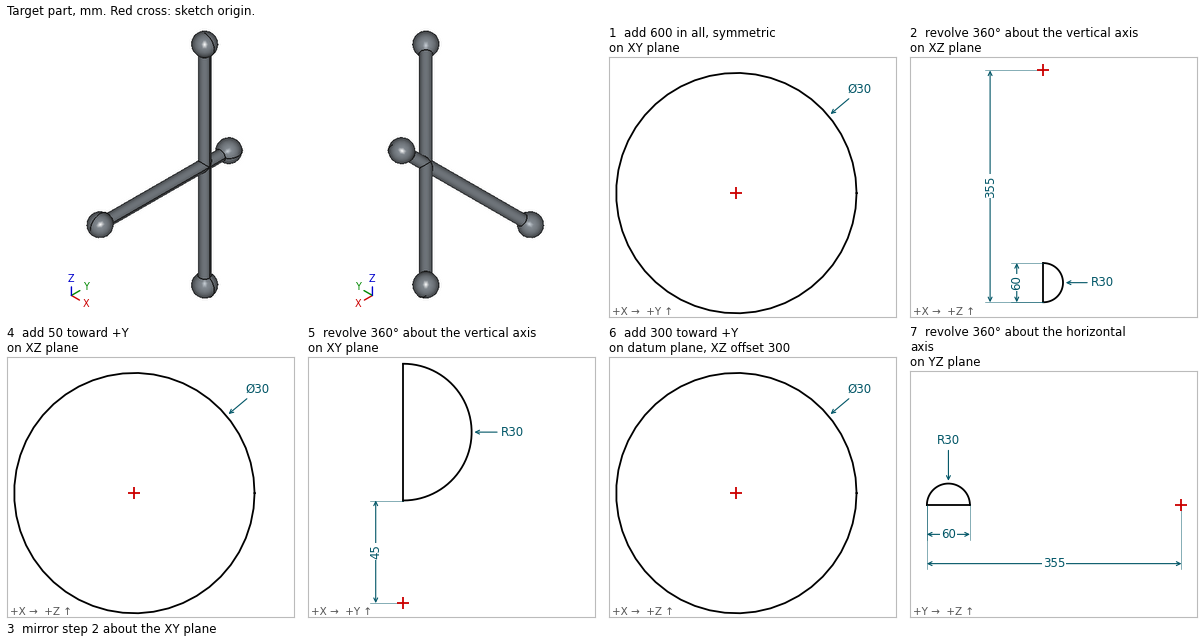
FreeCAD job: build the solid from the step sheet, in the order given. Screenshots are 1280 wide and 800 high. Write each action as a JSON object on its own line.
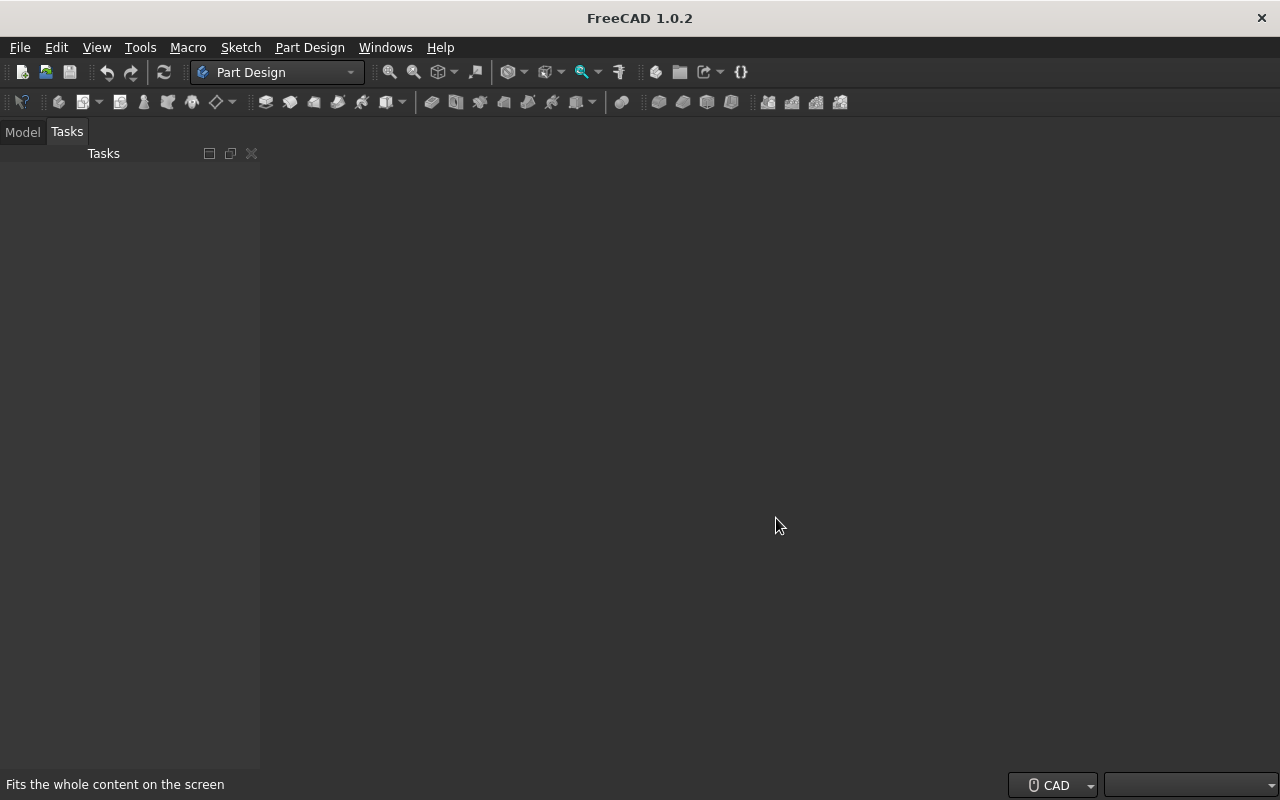
{"action": "key", "text": "ctrl+n"}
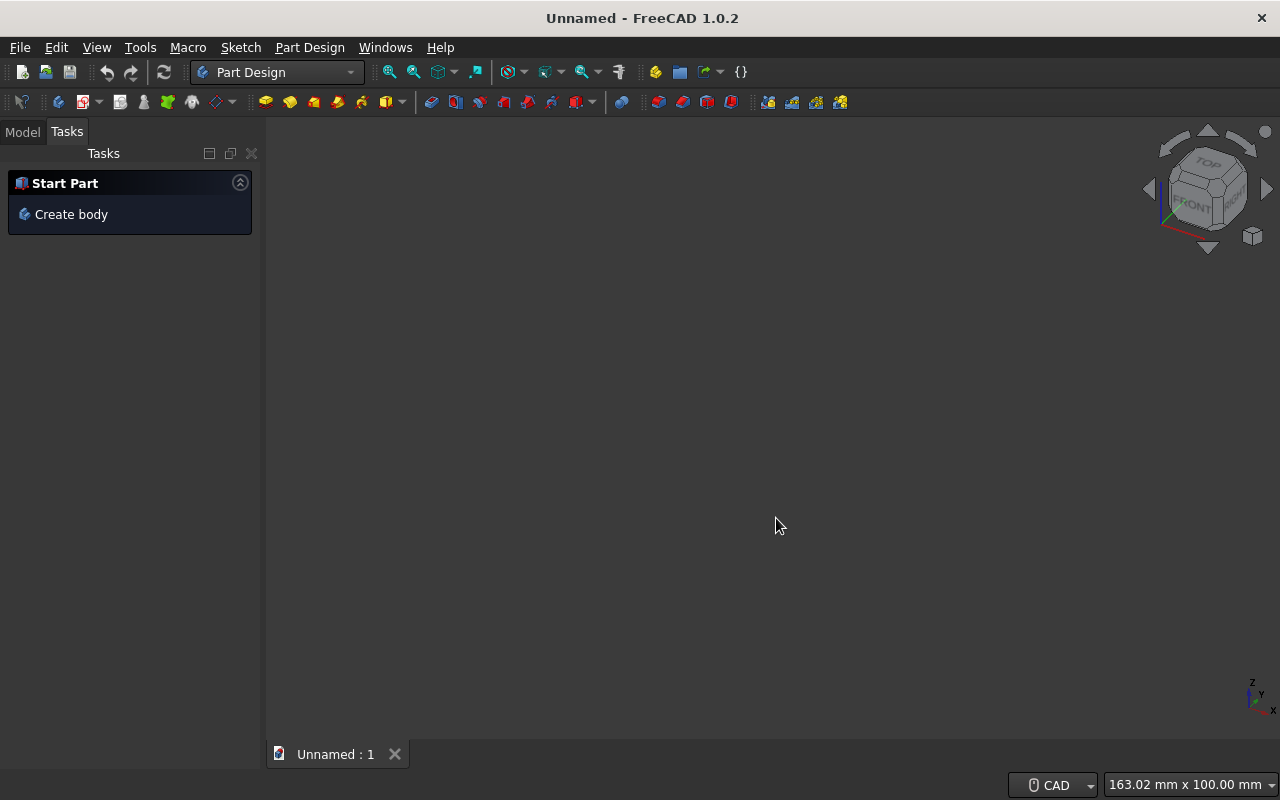
{"action": "left_click", "coordinate": [84, 102]}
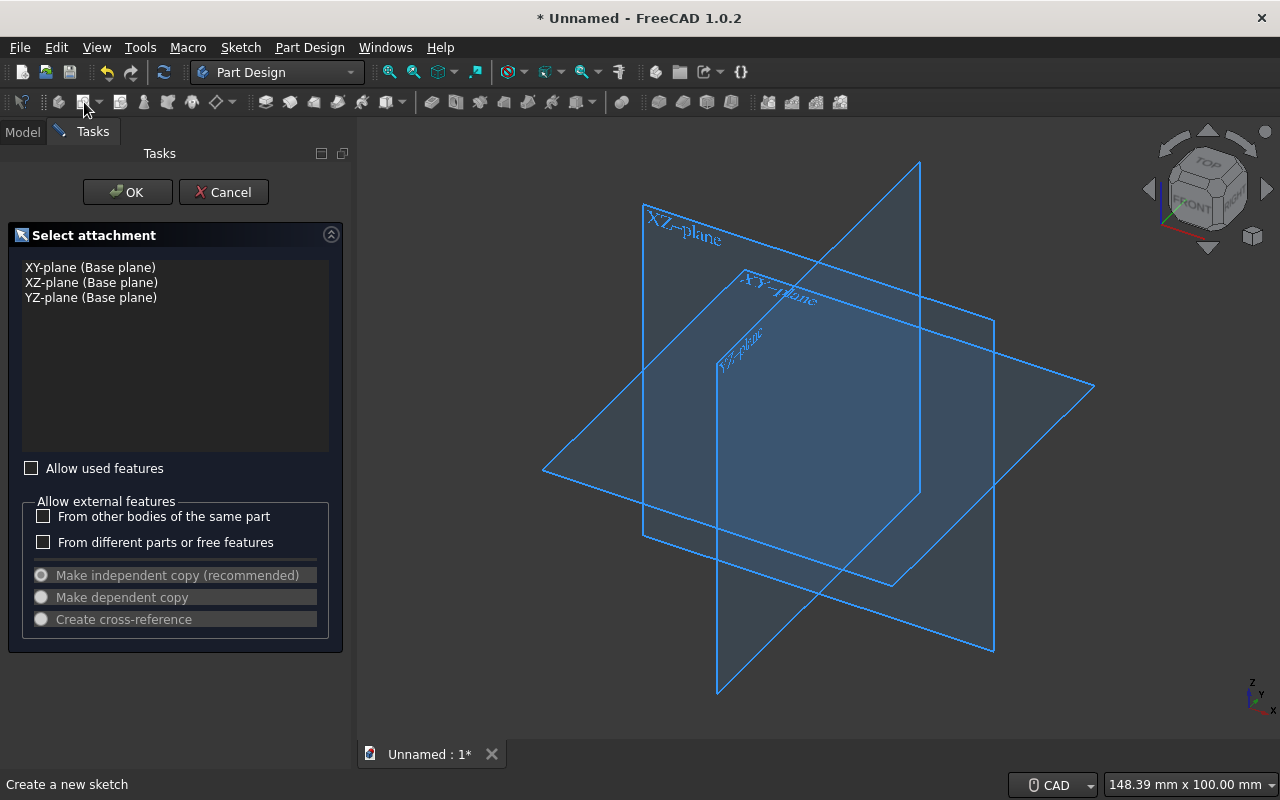
{"action": "left_click", "coordinate": [82, 268]}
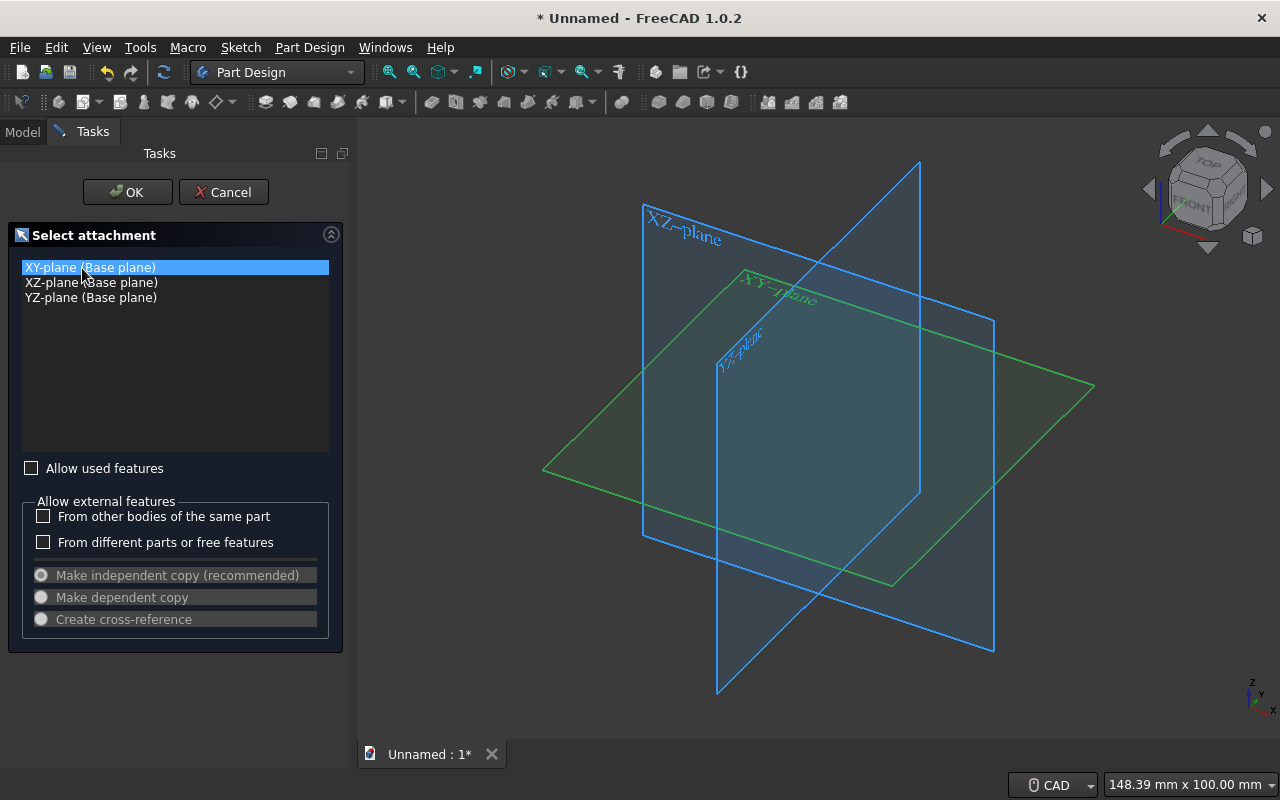
{"action": "left_click", "coordinate": [128, 192]}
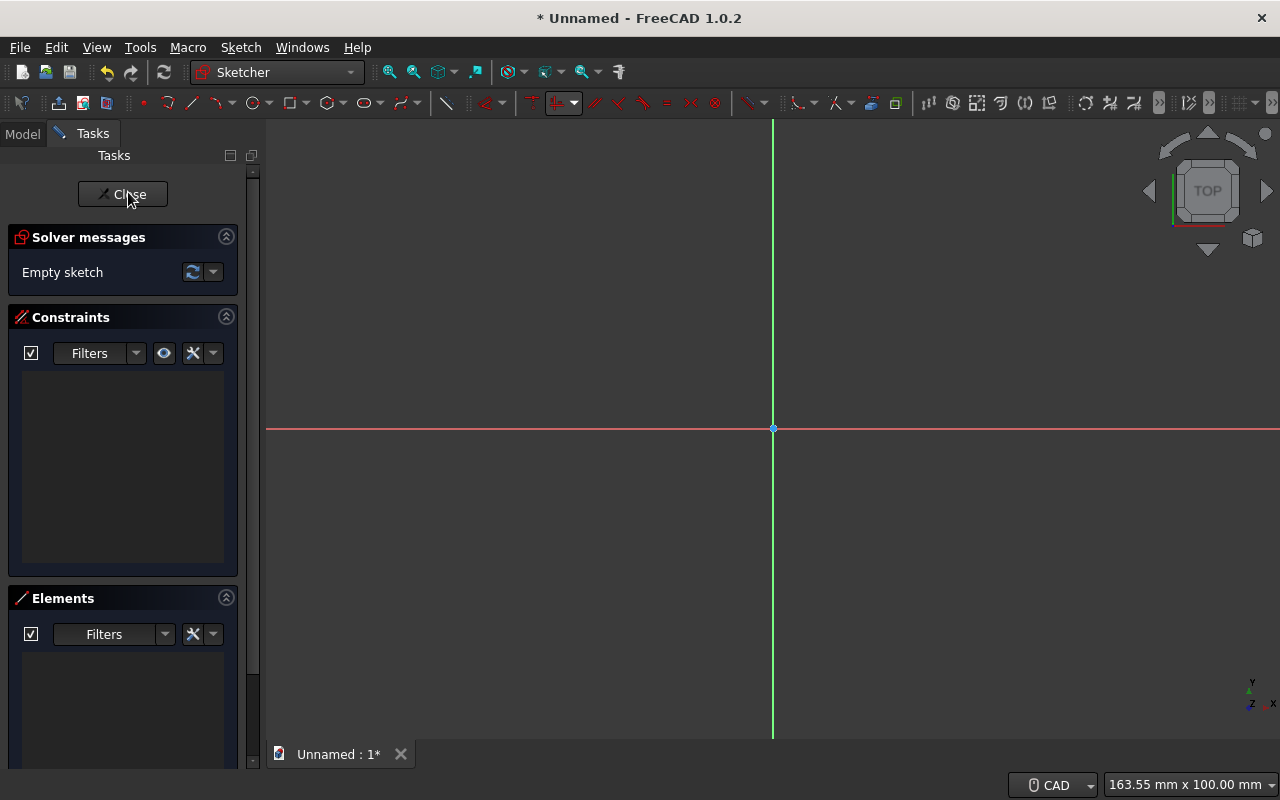
{"action": "scroll", "coordinate": [829, 429], "scroll_direction": "up", "scroll_amount": 4}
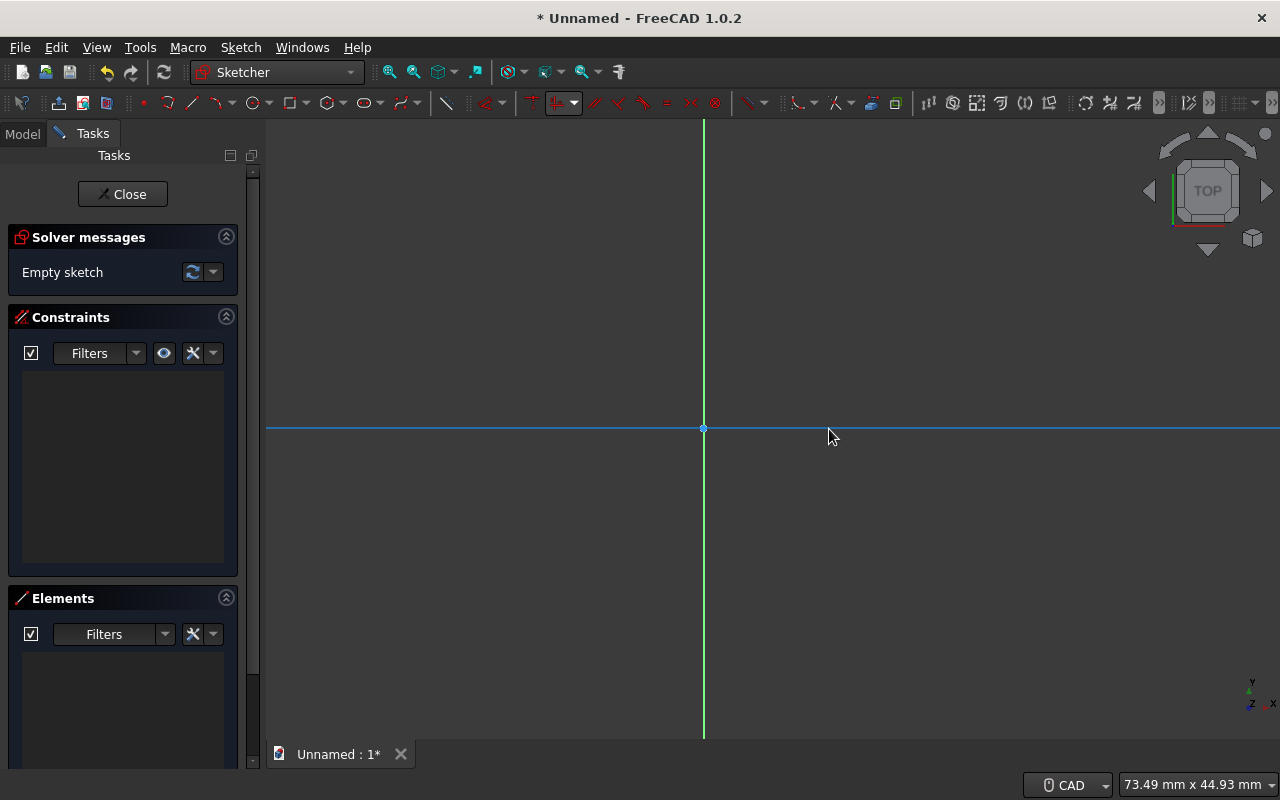
{"action": "left_click", "coordinate": [254, 104]}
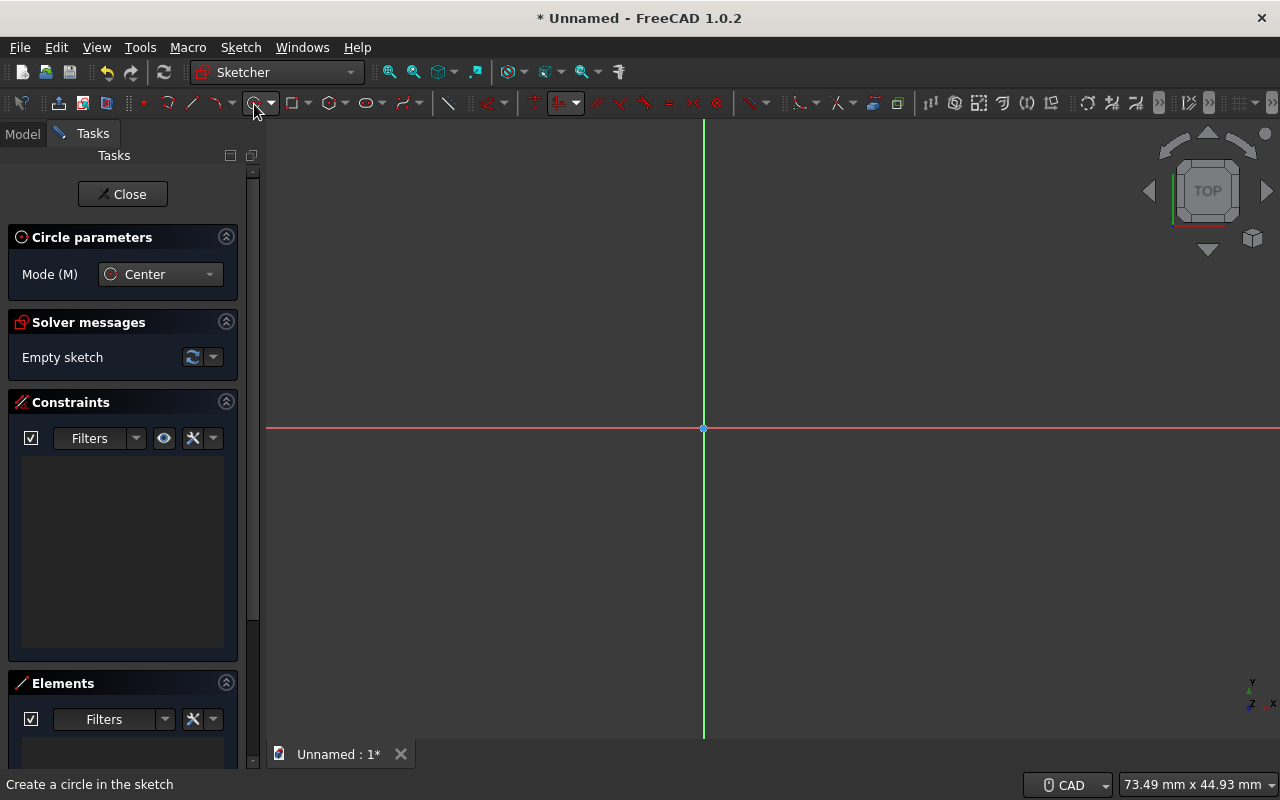
{"action": "left_click", "coordinate": [704, 428]}
{"action": "left_click", "coordinate": [850, 282]}
{"action": "key", "text": "Escape"}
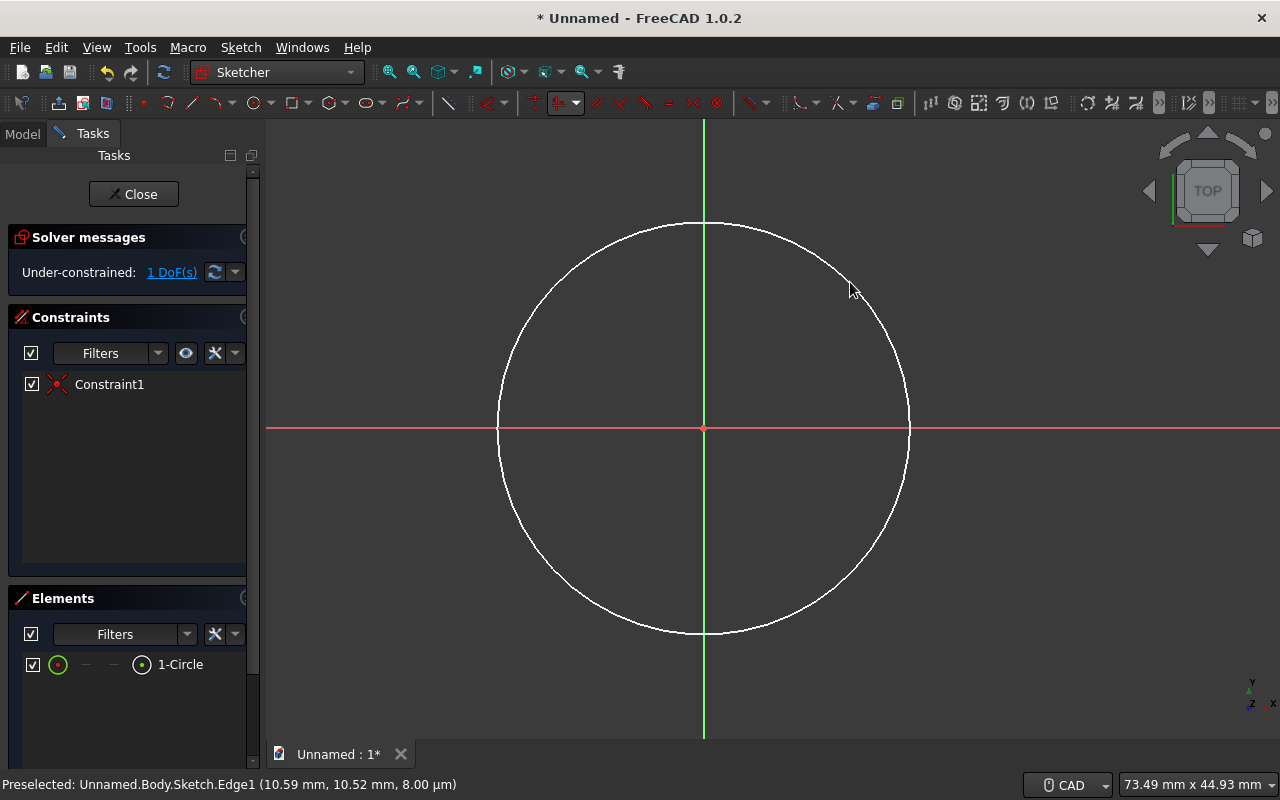
{"action": "left_click", "coordinate": [849, 282]}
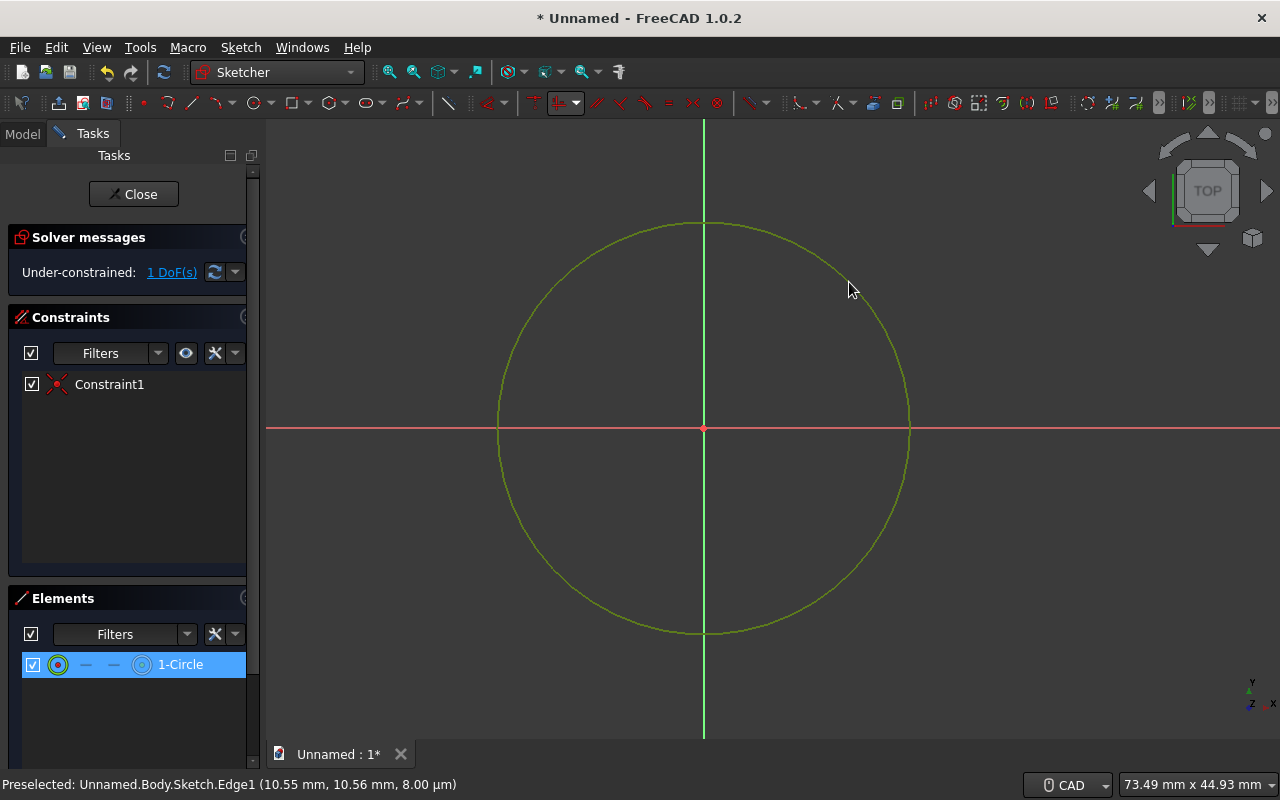
{"action": "key", "text": "k o"}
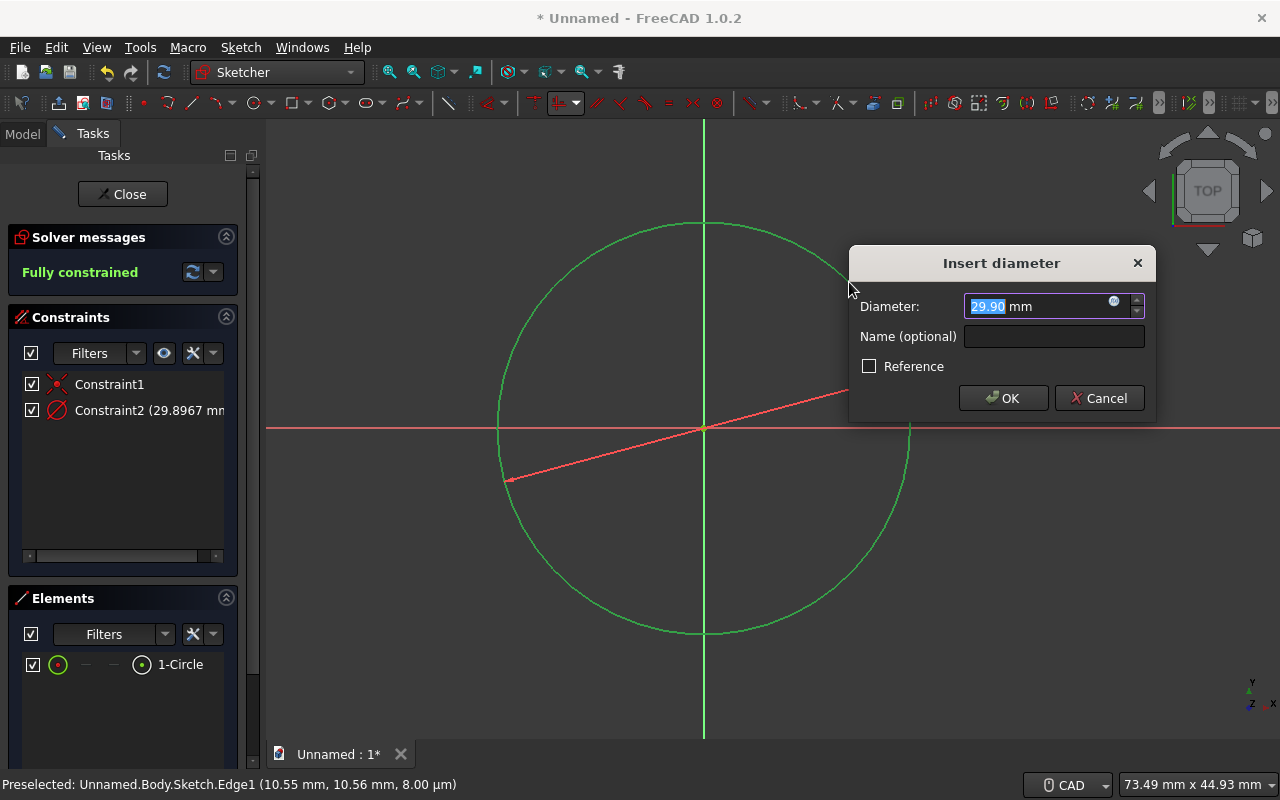
{"action": "type", "text": "30"}
{"action": "key", "text": "Return"}